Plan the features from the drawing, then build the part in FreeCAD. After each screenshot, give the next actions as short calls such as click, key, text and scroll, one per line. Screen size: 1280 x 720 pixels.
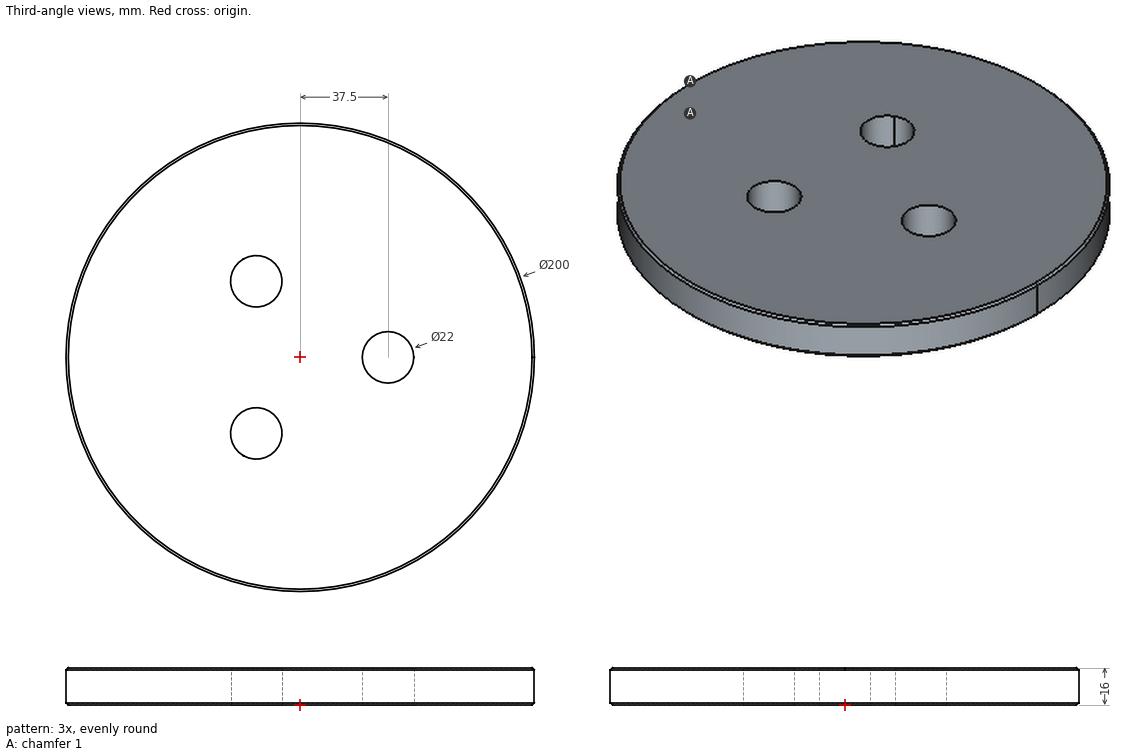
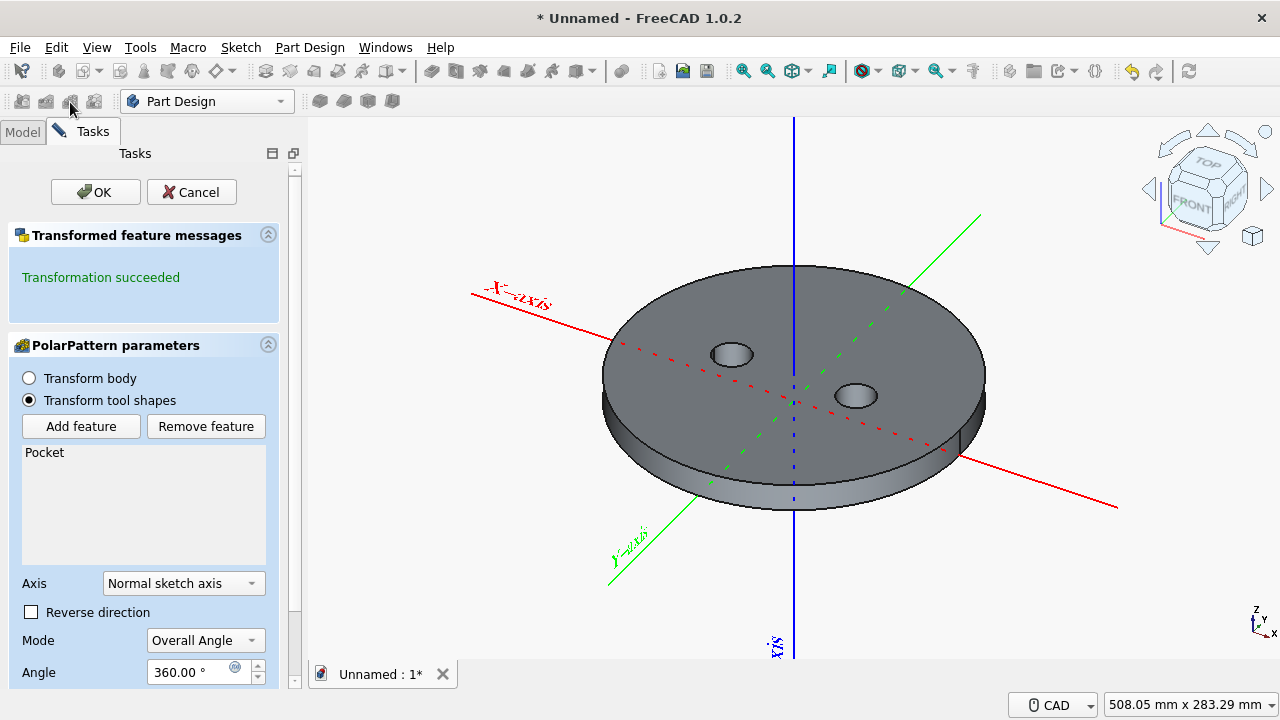
click(184, 584)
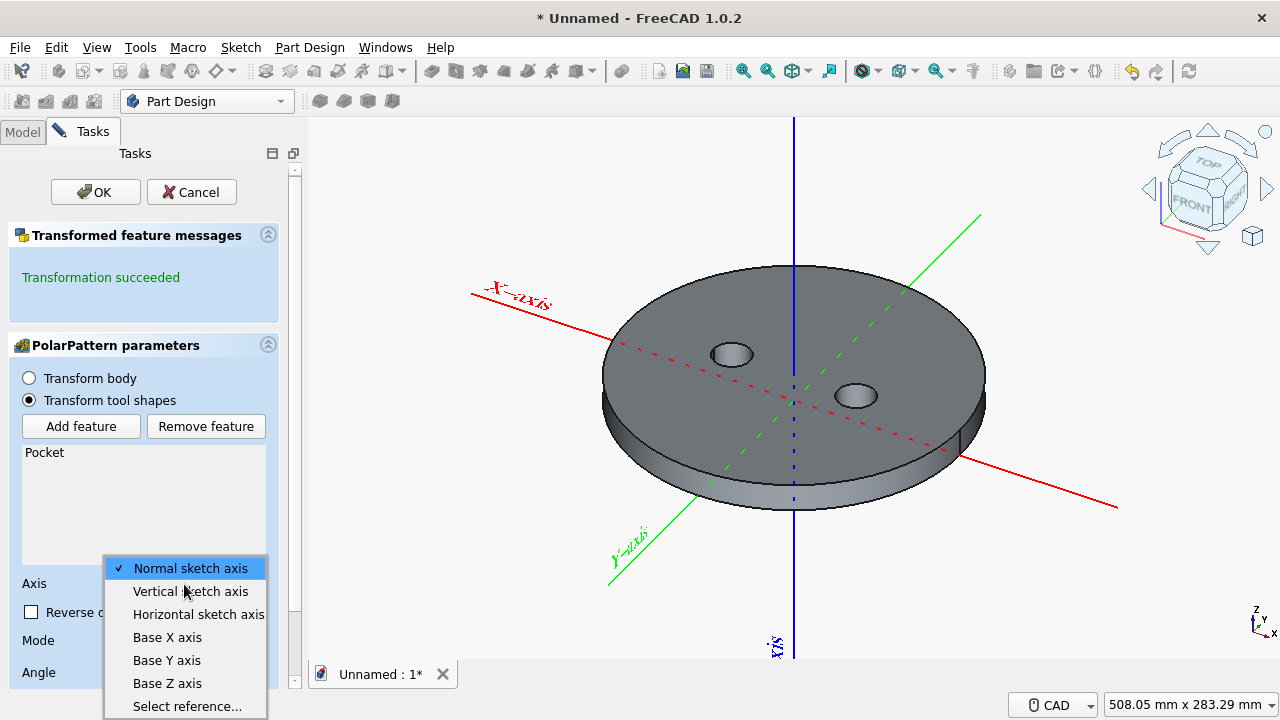
click(184, 684)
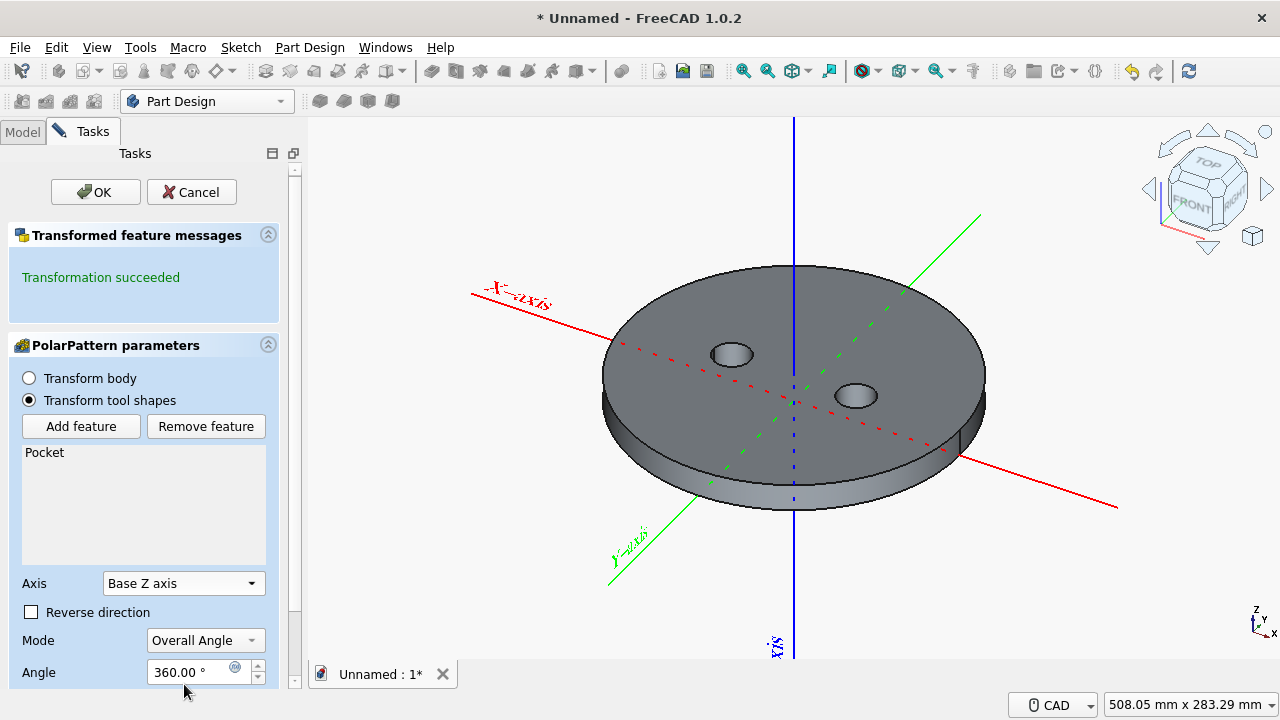
scroll(295, 426, down, 2)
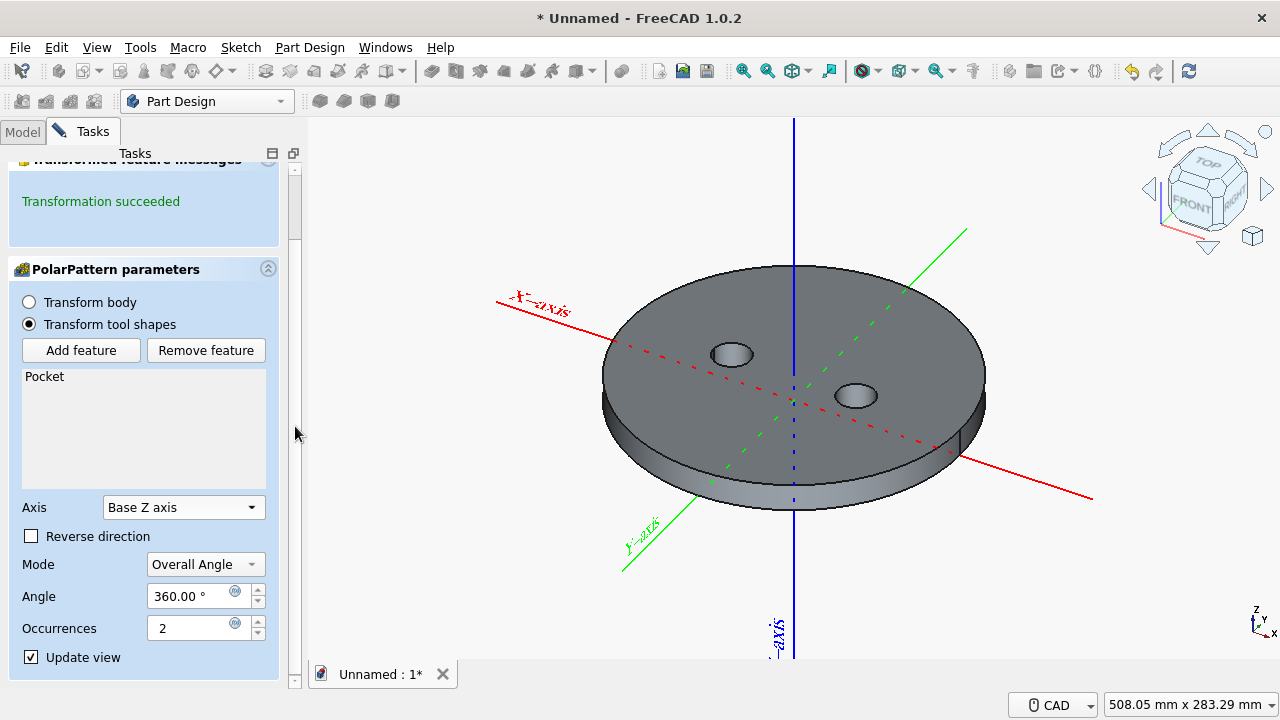
triple_click(198, 628)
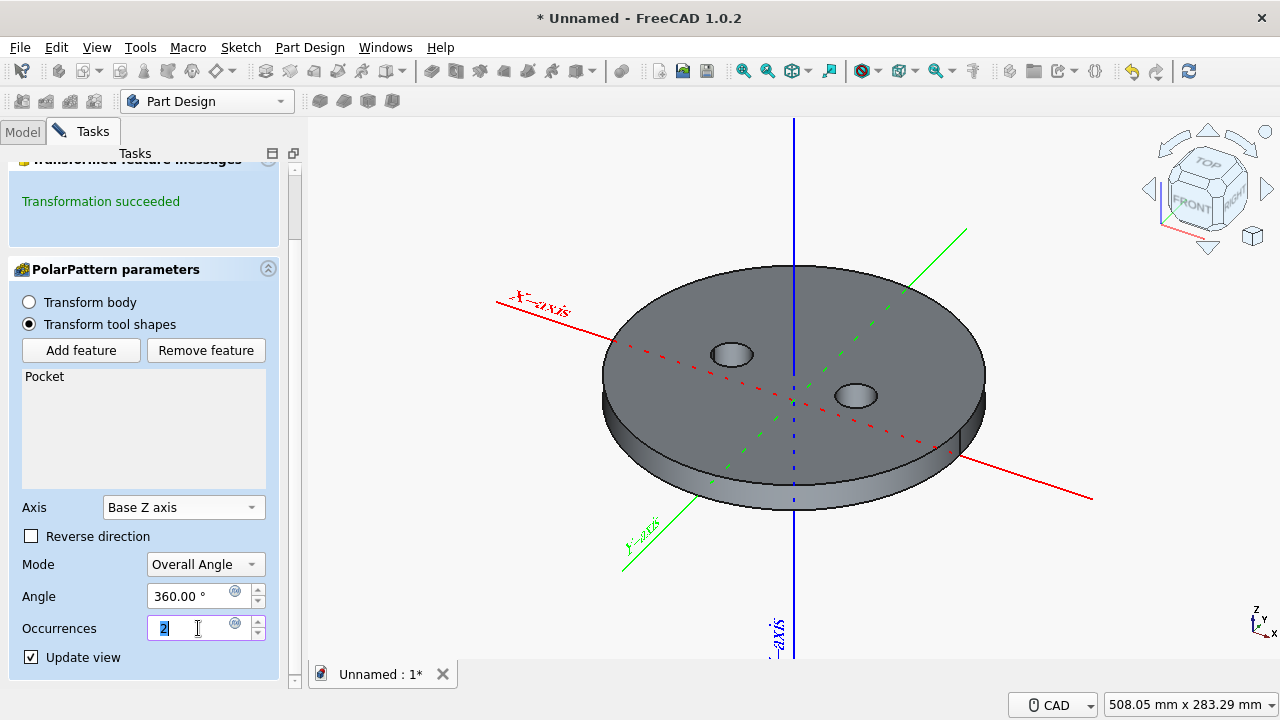
text(3)
key(Tab)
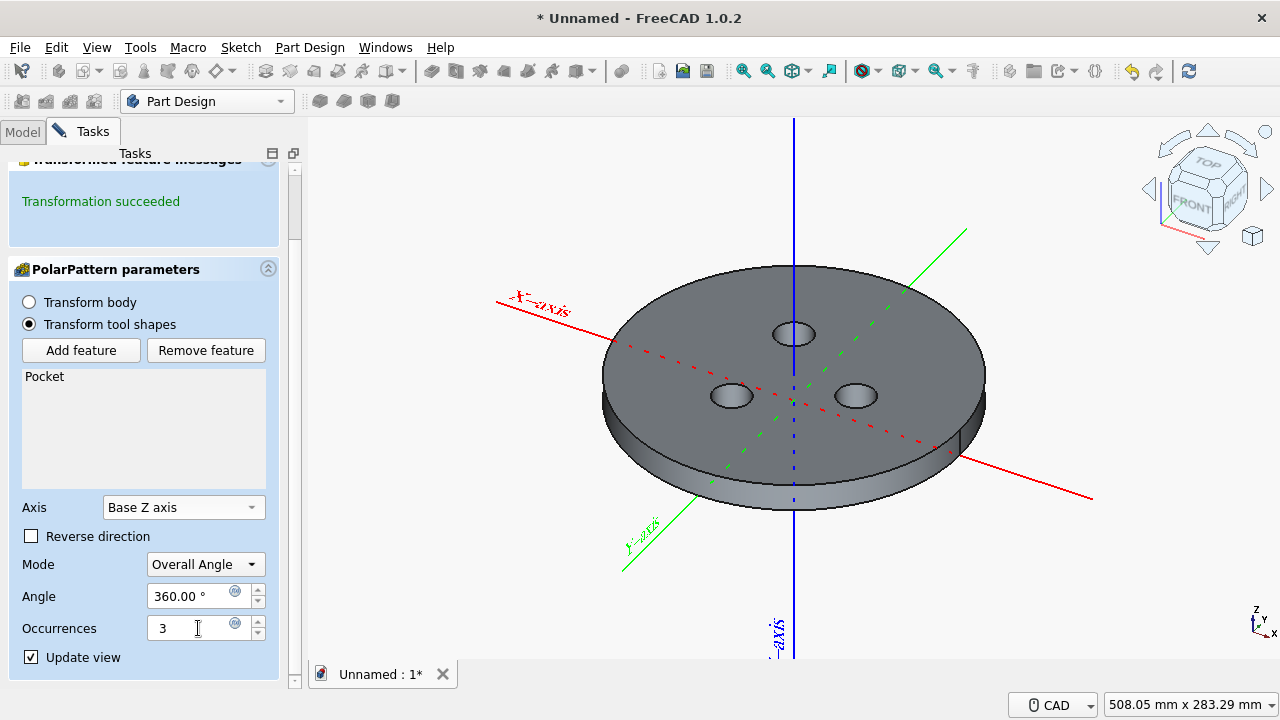
scroll(295, 426, up, 3)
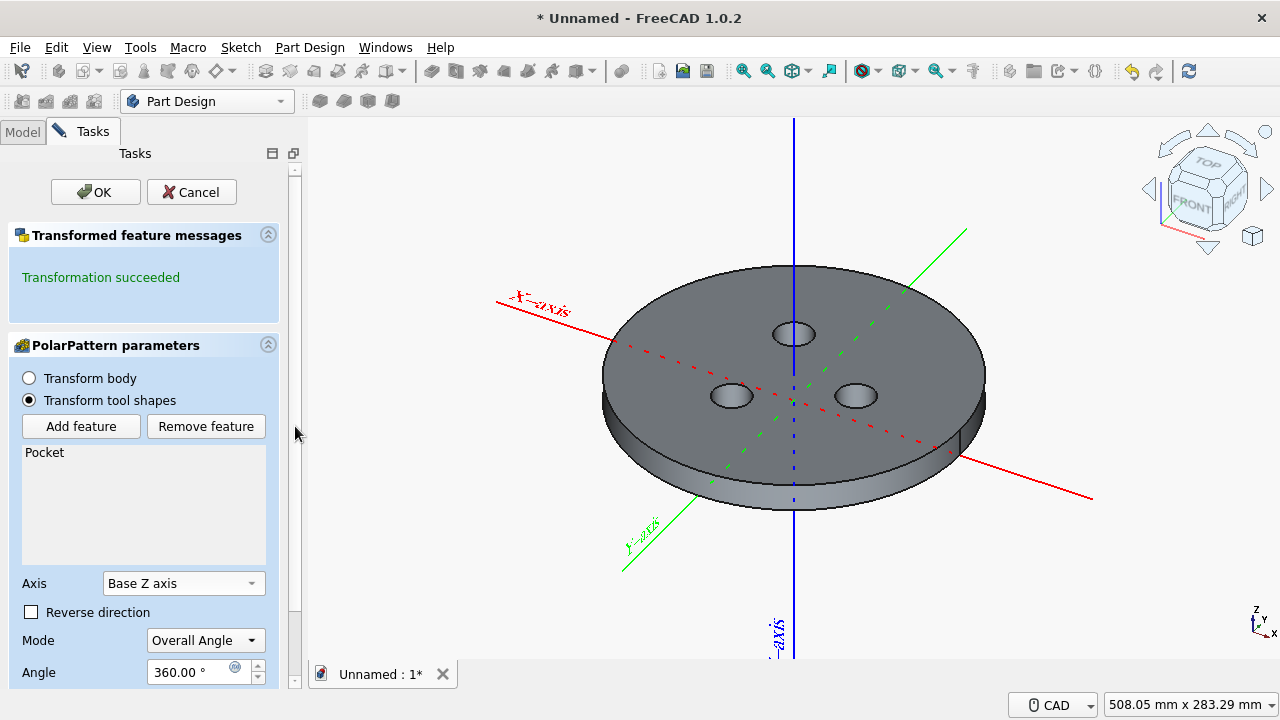
click(96, 192)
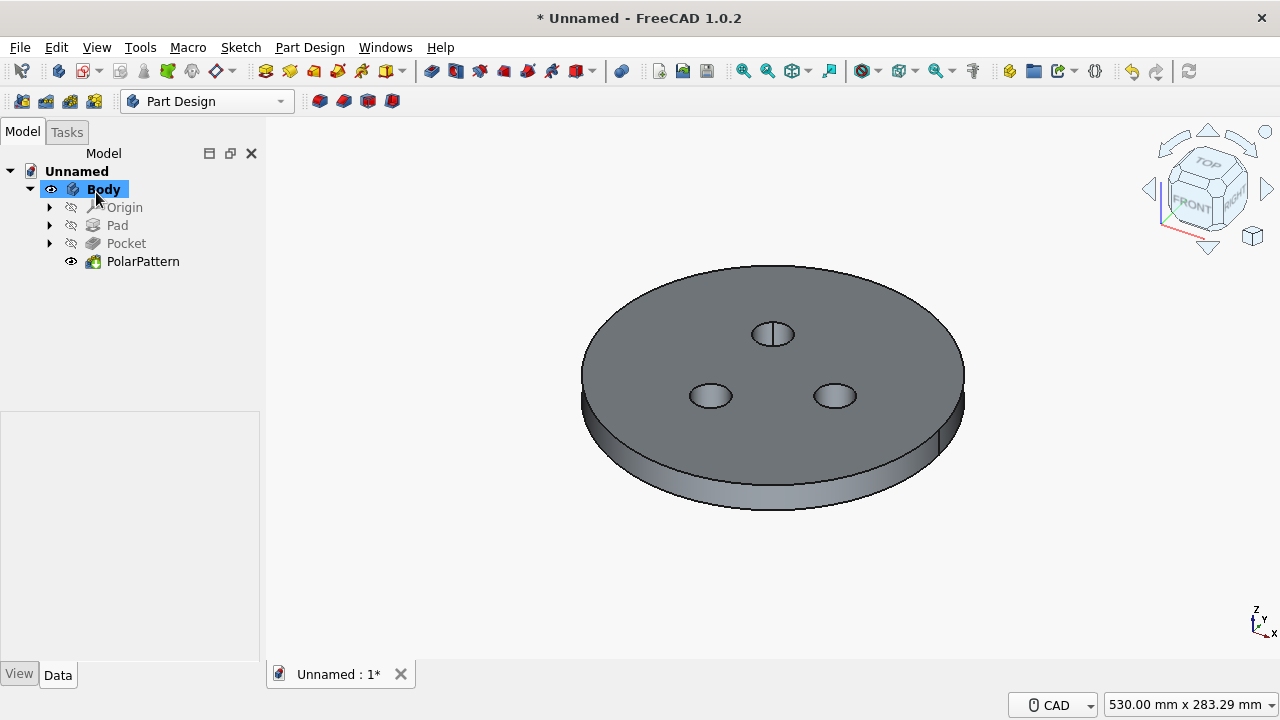
click(583, 386)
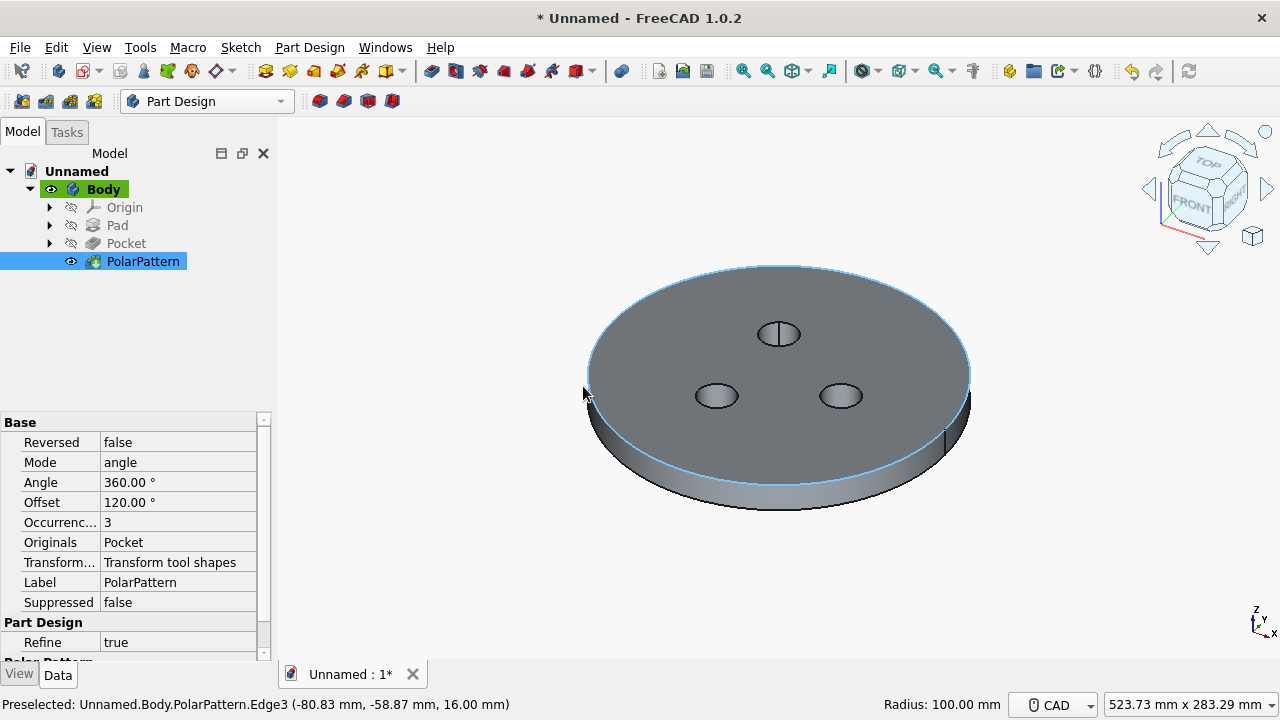
key(0)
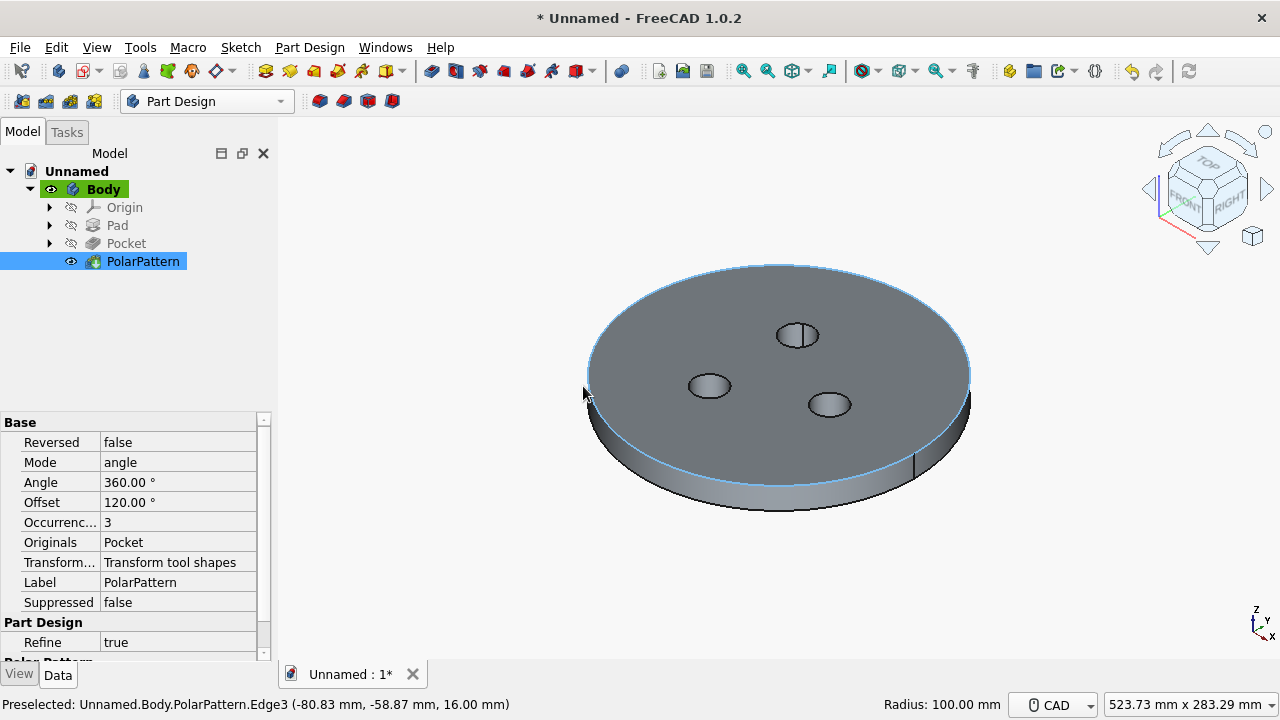
key(2)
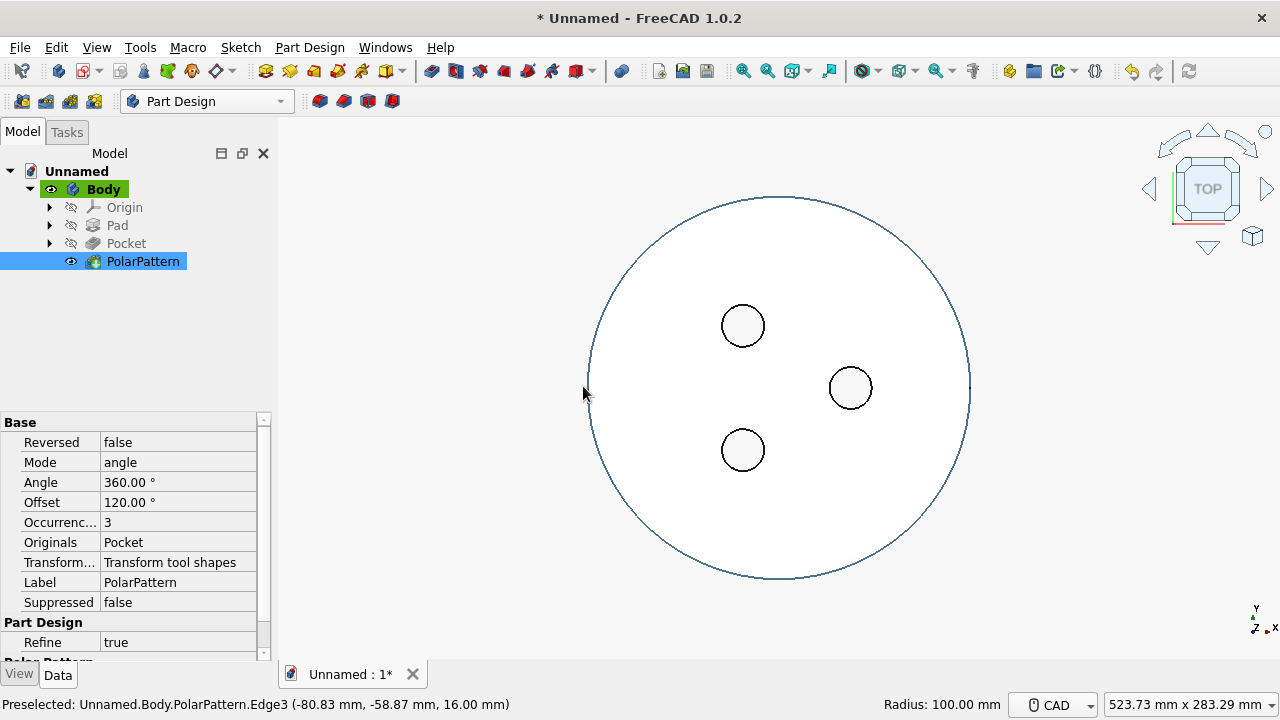
key(1)